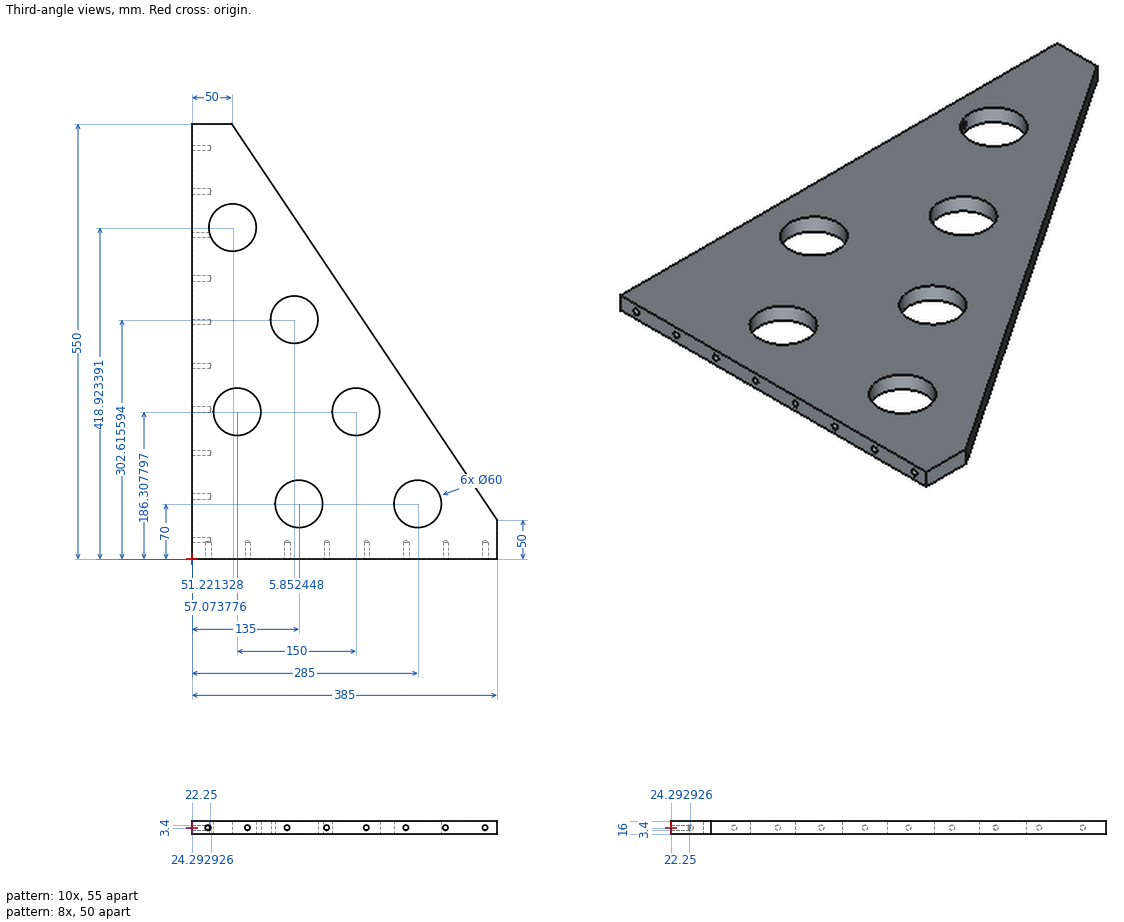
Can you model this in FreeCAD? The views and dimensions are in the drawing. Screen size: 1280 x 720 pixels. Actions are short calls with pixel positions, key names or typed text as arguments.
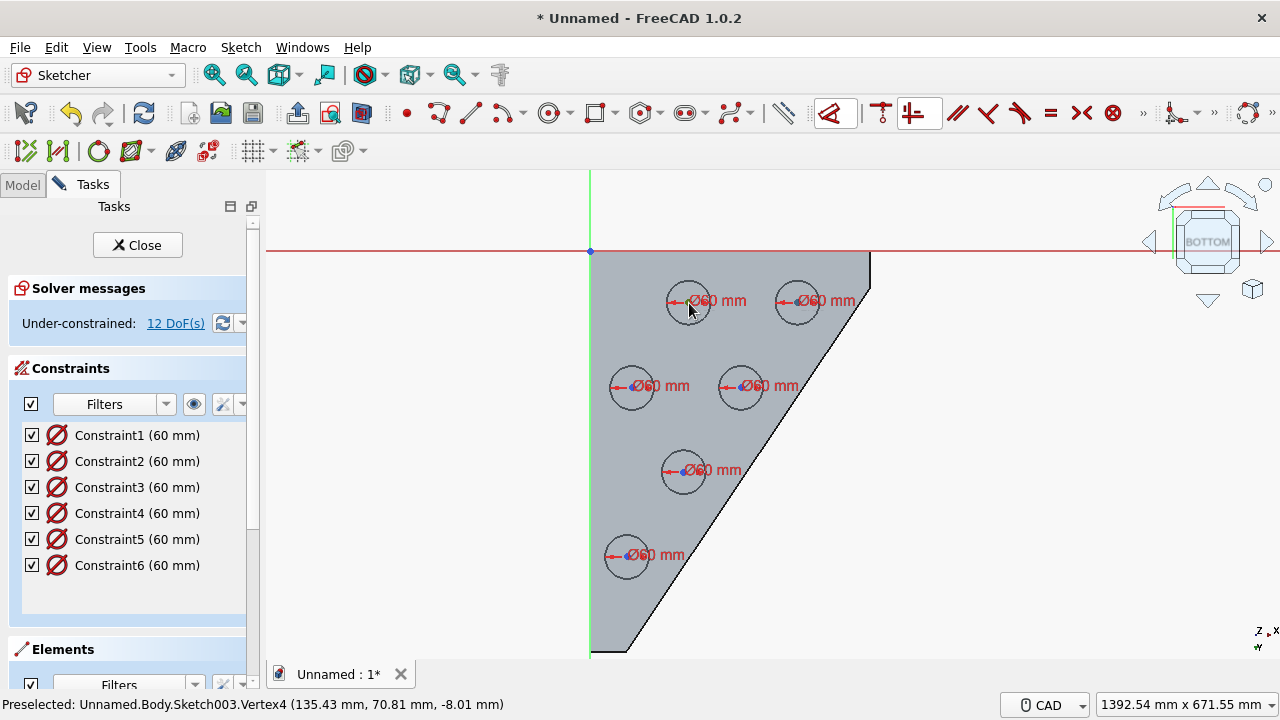
click(936, 114)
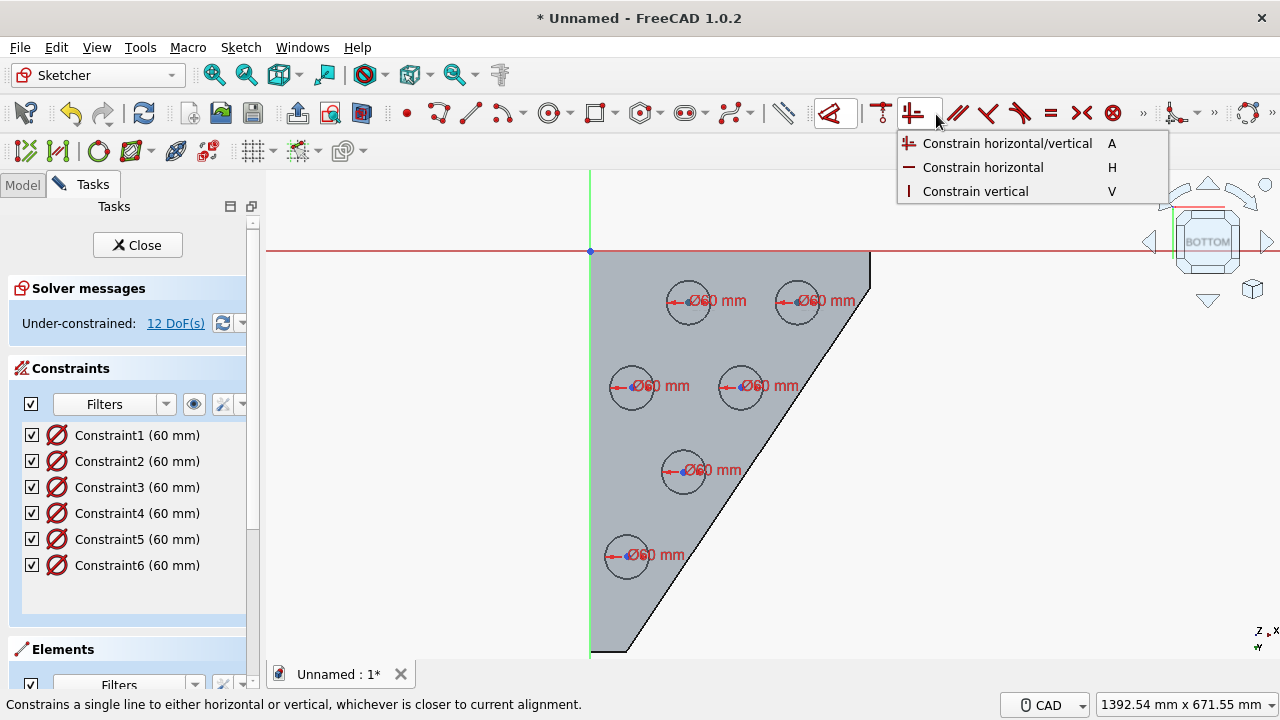
click(1033, 167)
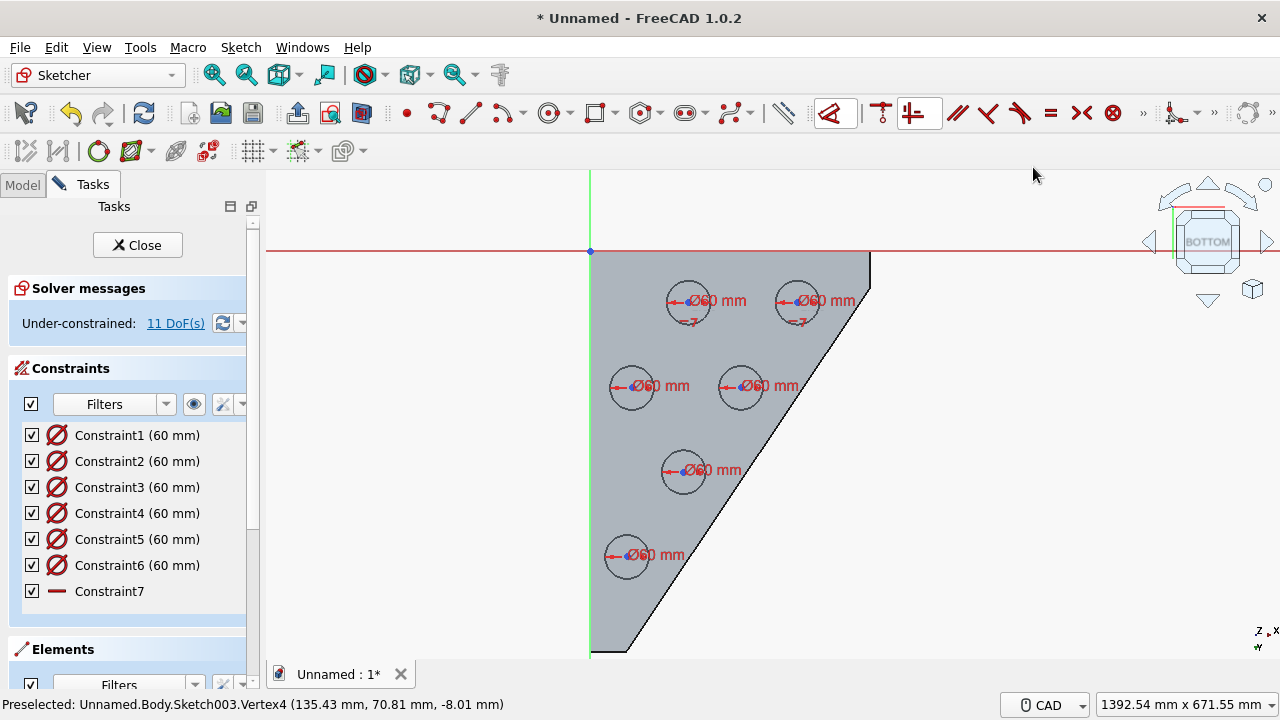
click(741, 388)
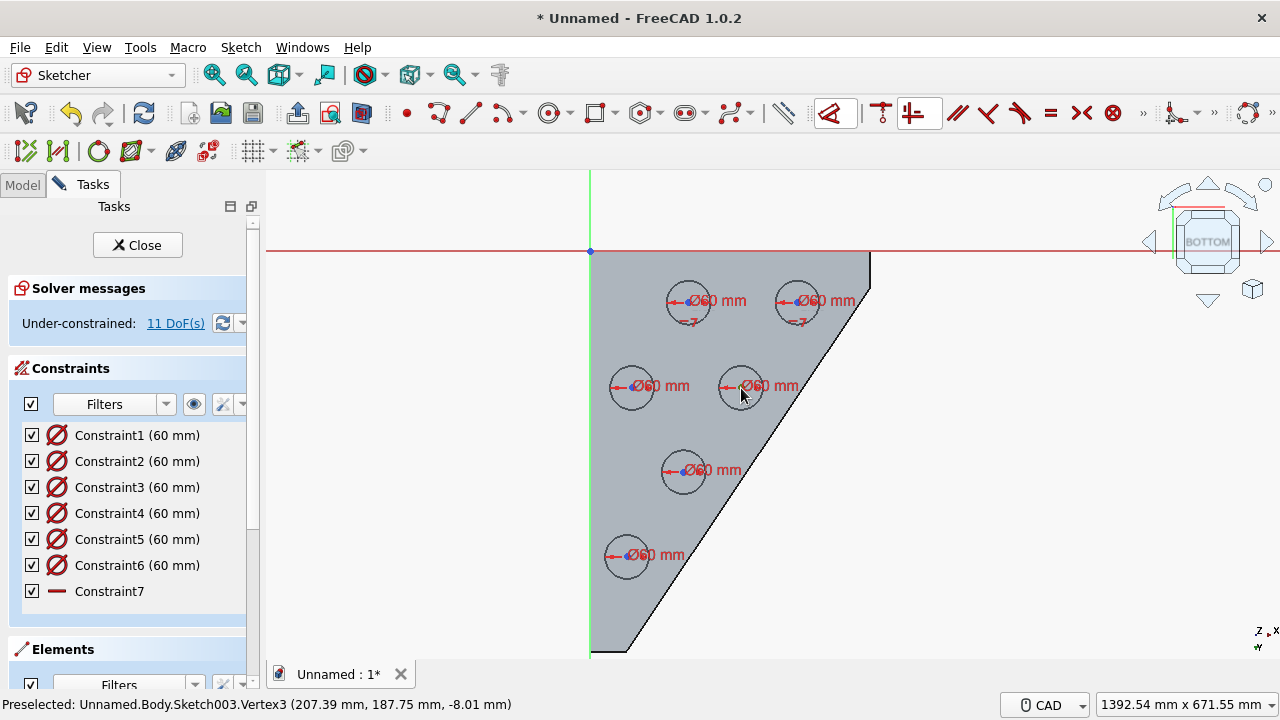
click(632, 388)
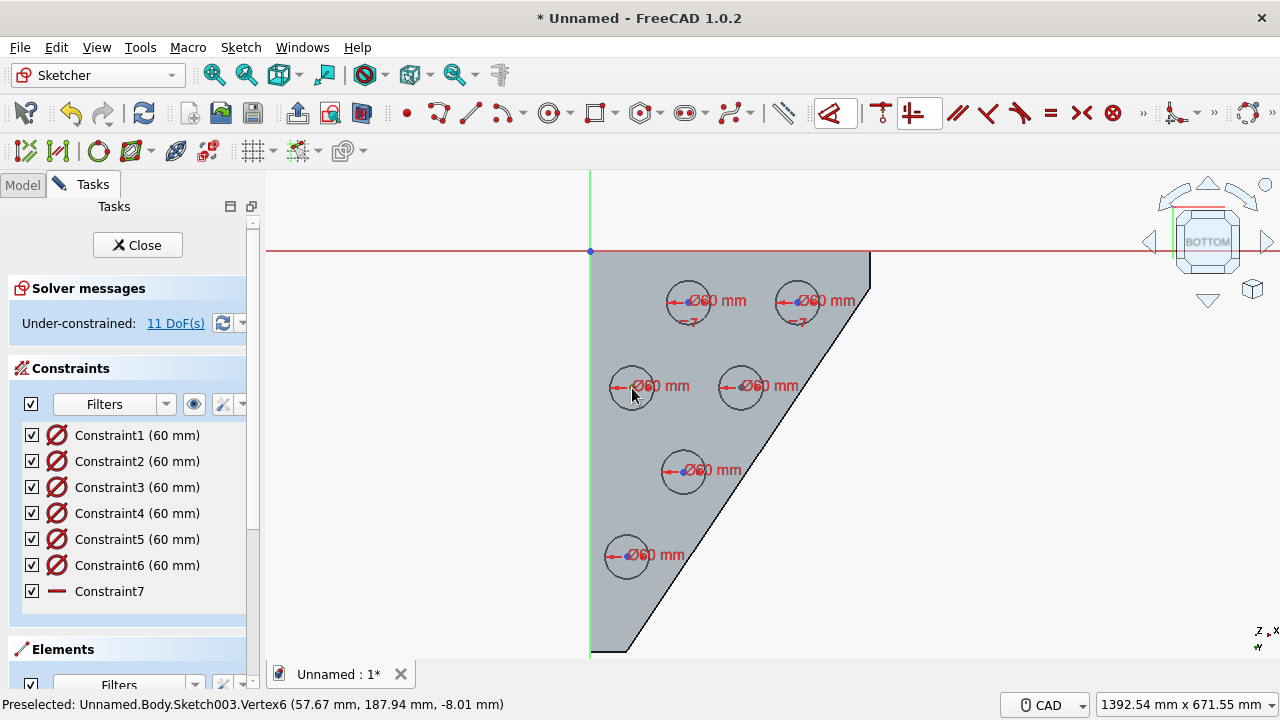
click(936, 114)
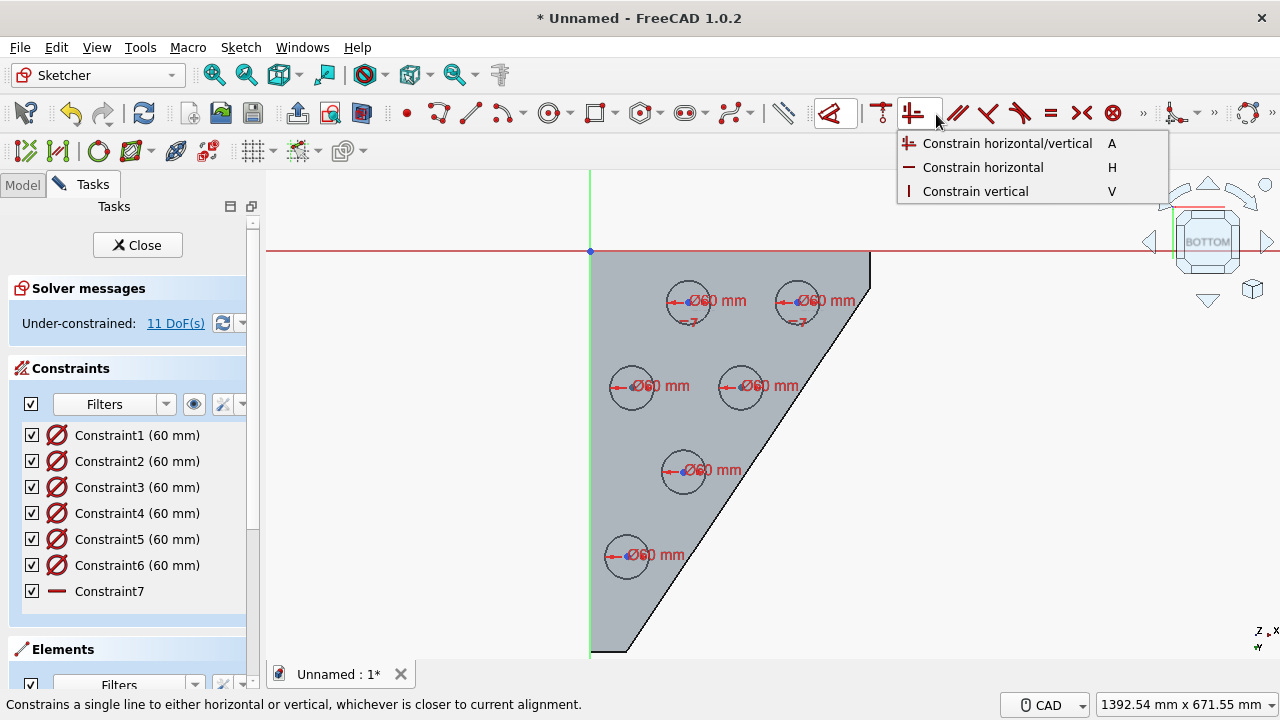
click(1033, 167)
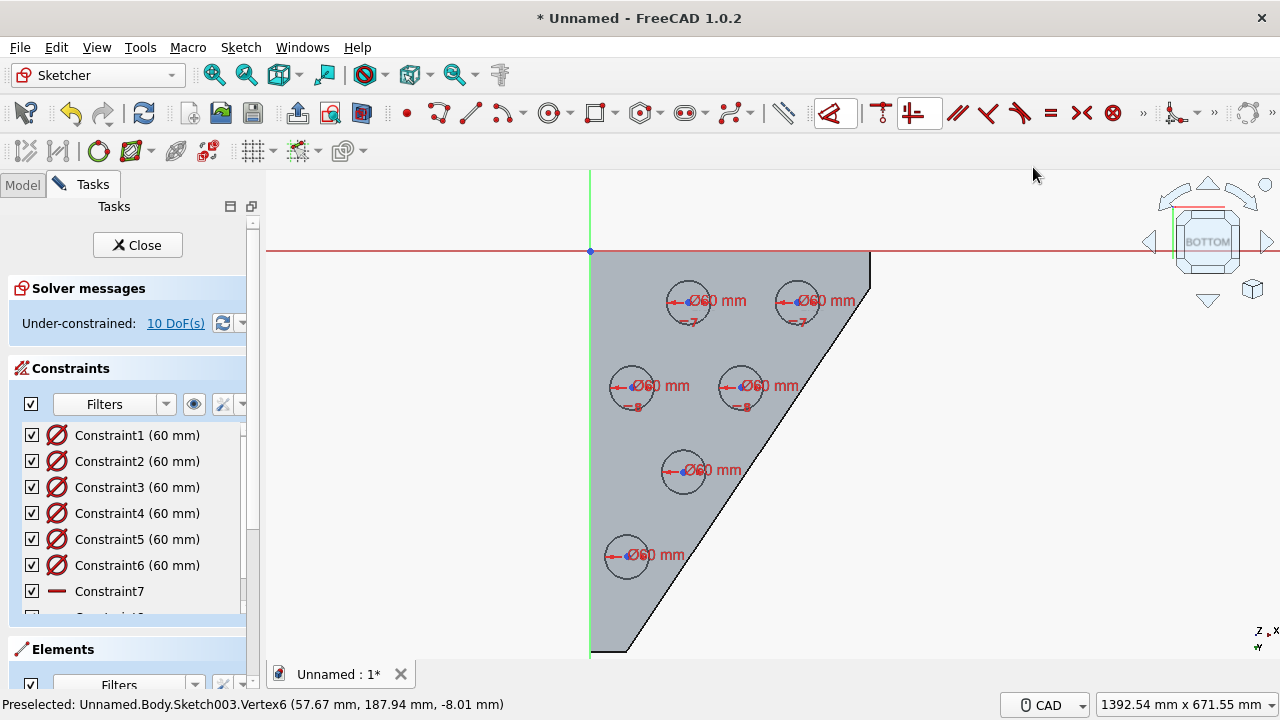
click(798, 303)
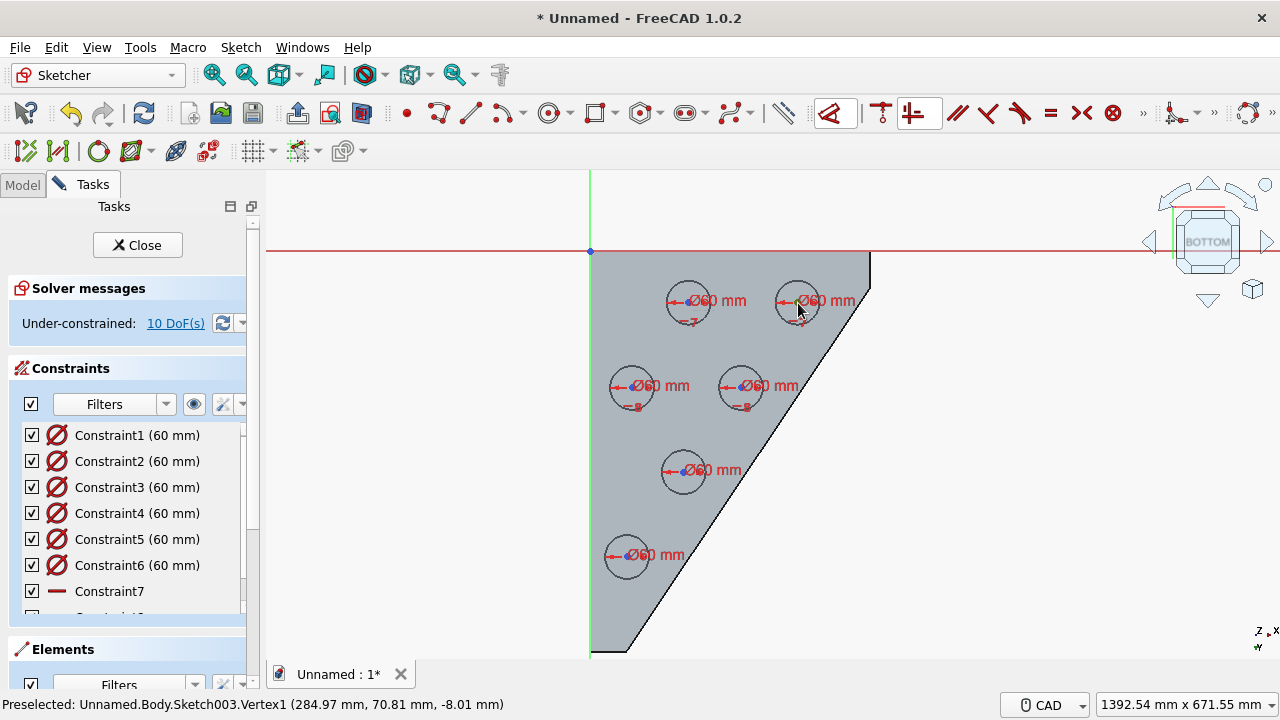
key(i)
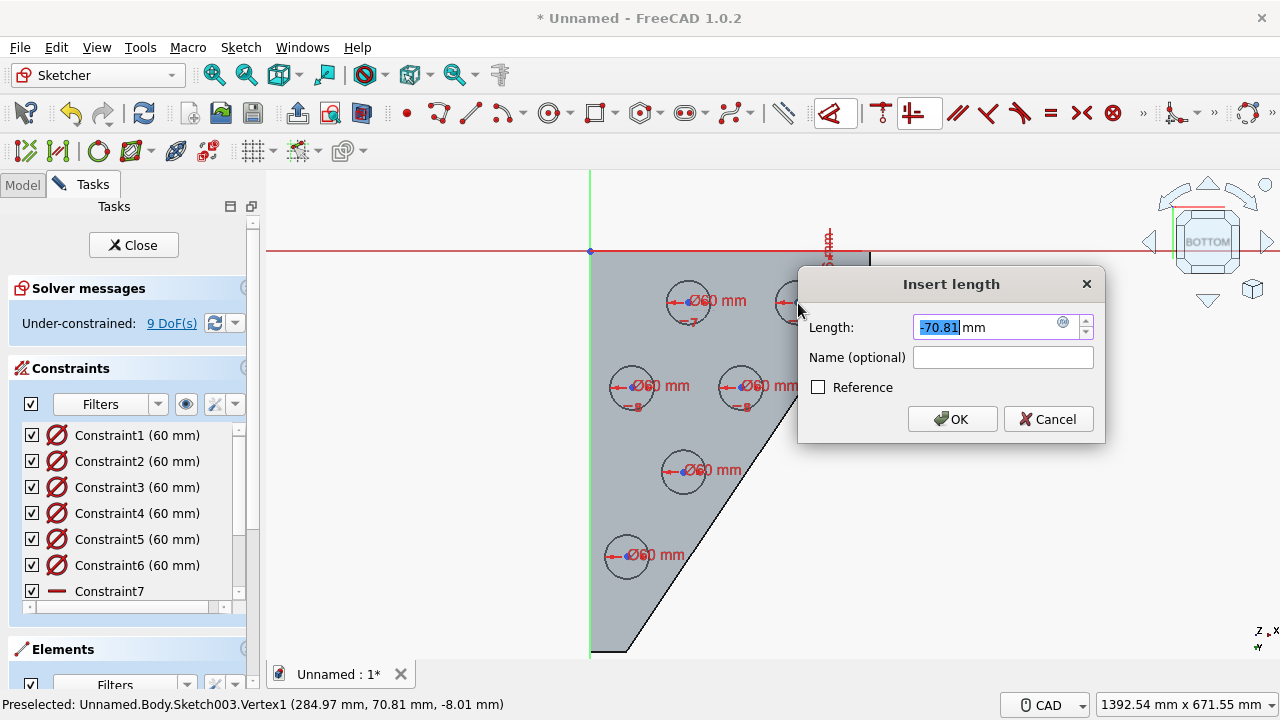
text(-70)
key(Return)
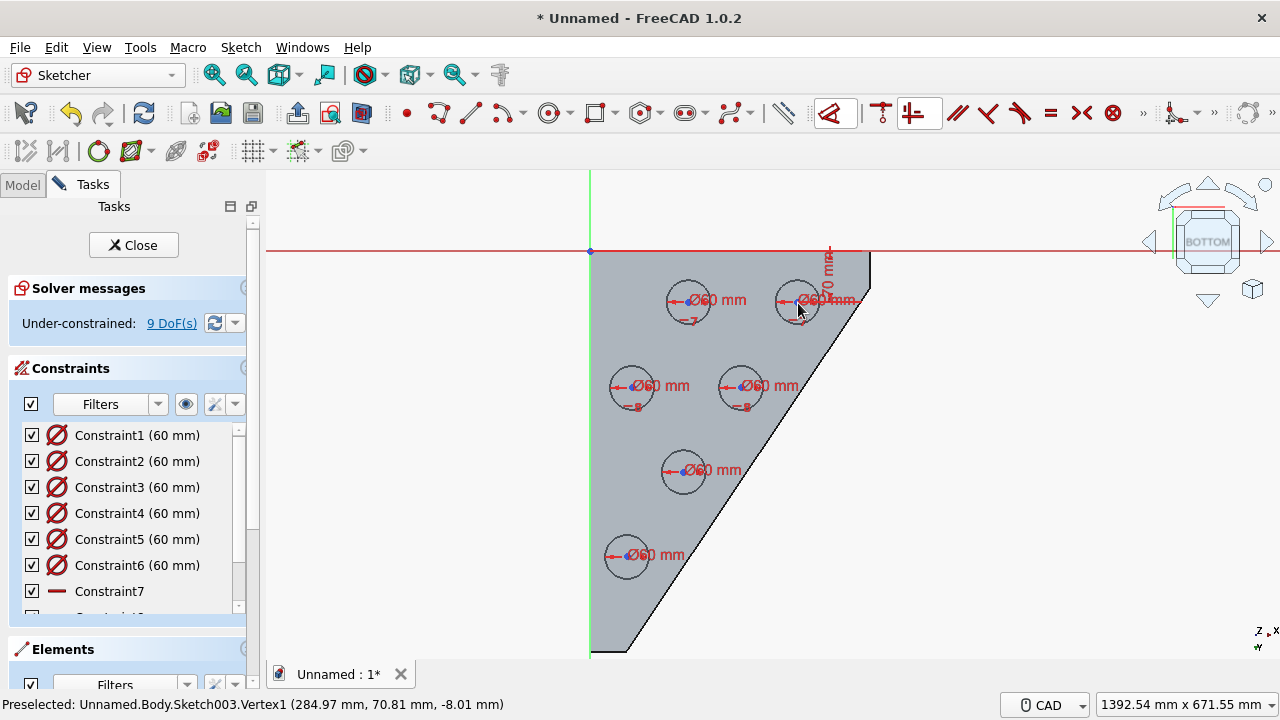
click(798, 302)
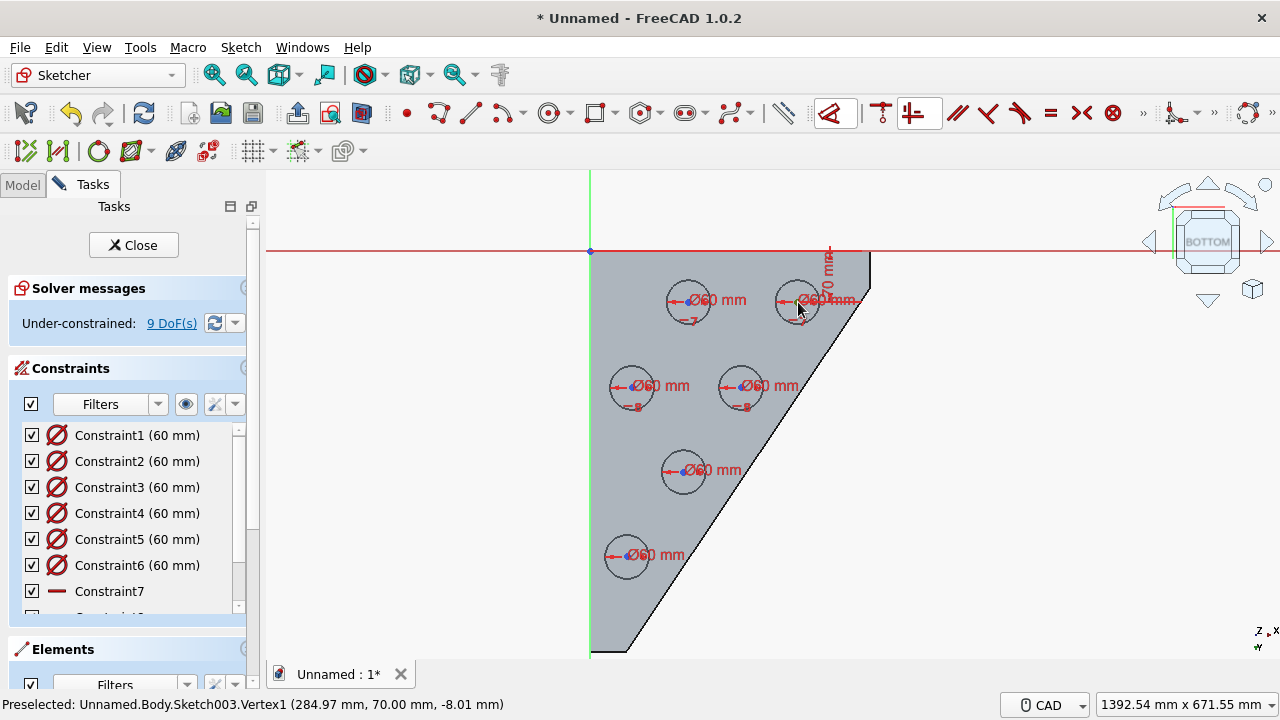
click(852, 114)